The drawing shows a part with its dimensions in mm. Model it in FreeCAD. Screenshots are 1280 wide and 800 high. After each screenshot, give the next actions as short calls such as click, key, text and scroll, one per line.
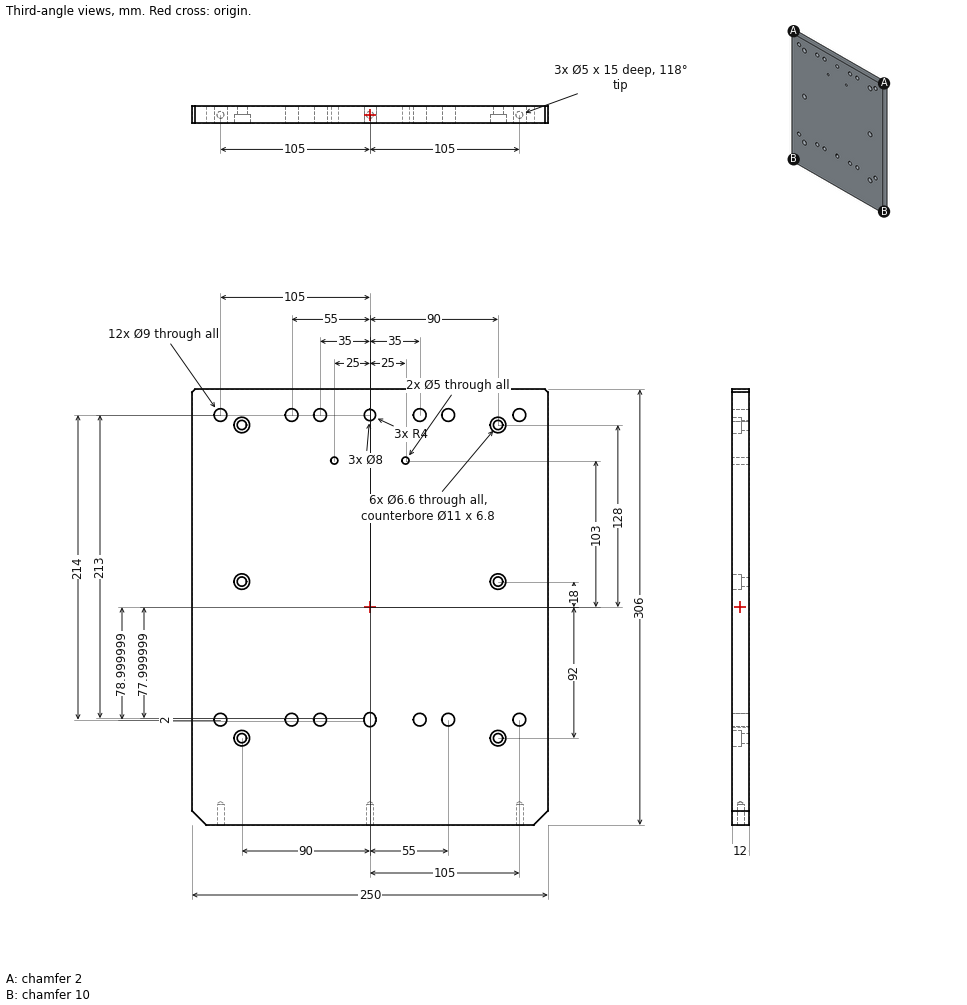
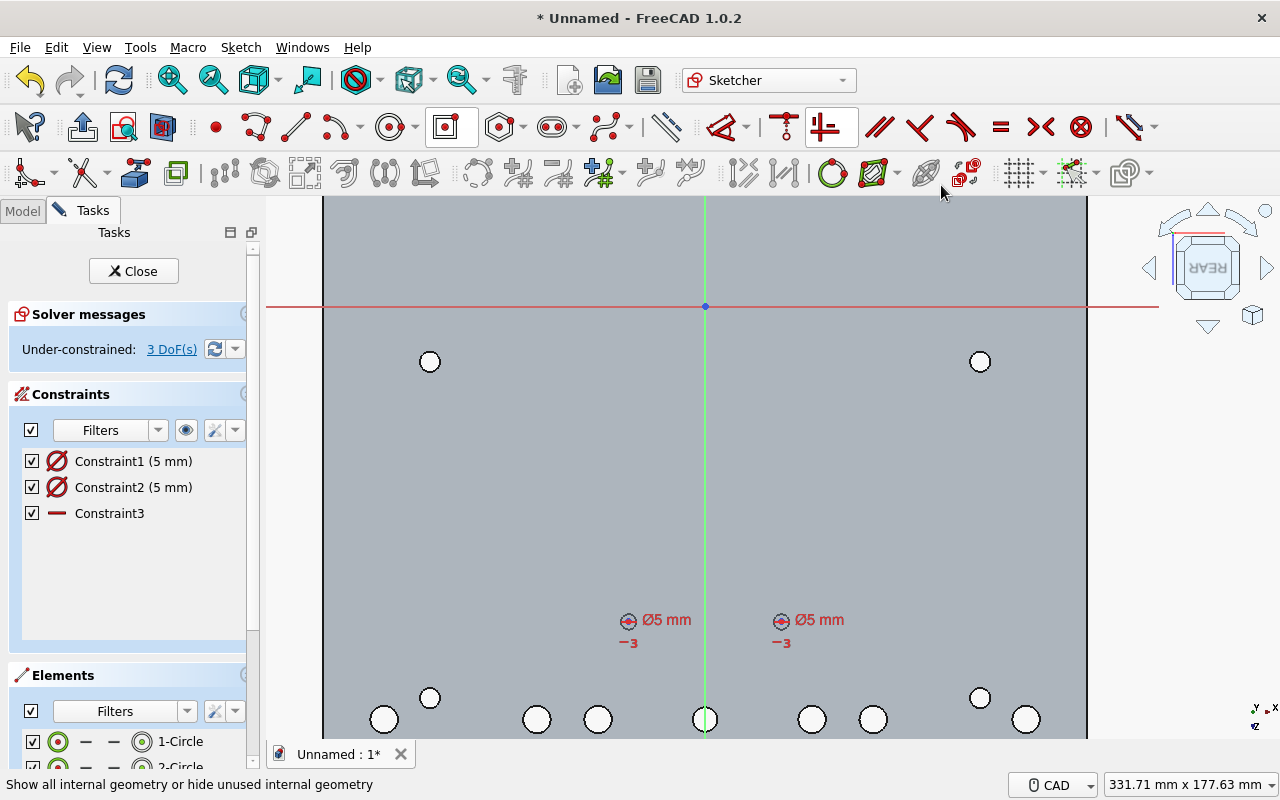
click(722, 128)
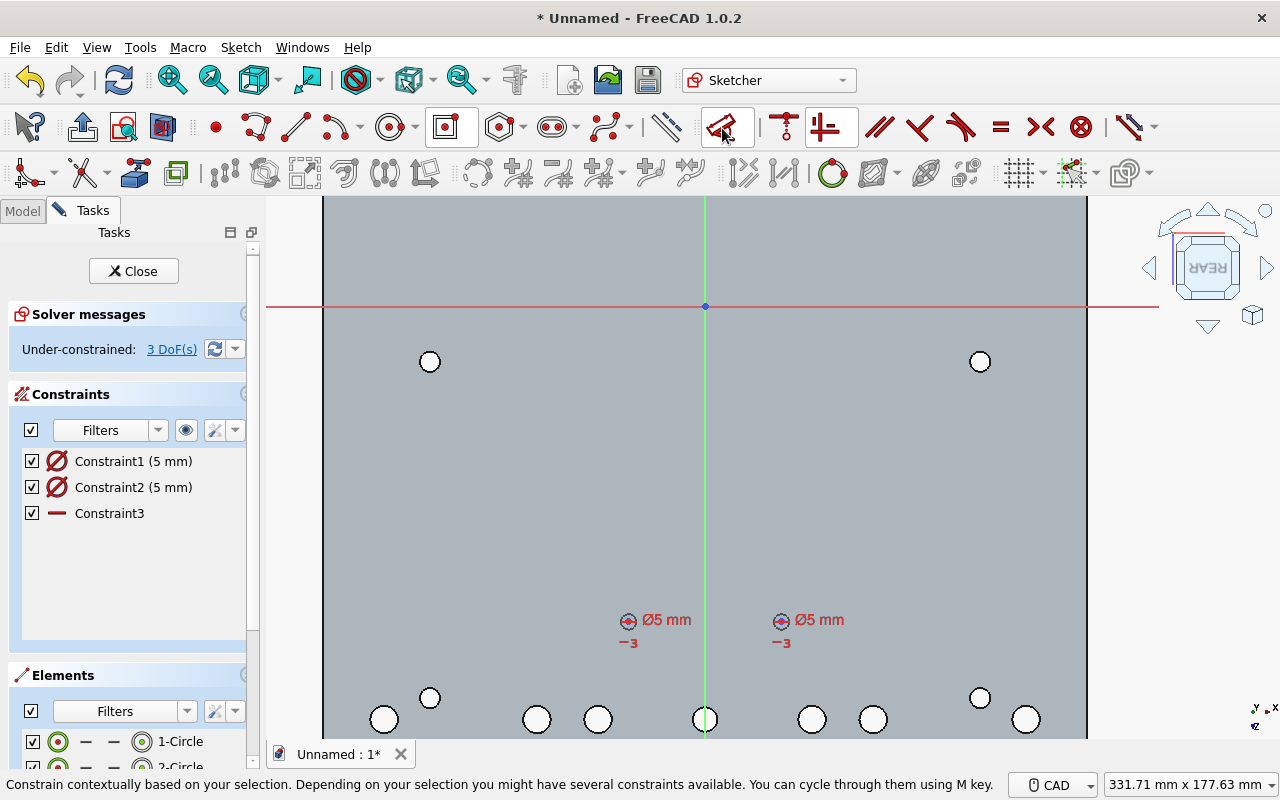
click(781, 622)
click(743, 273)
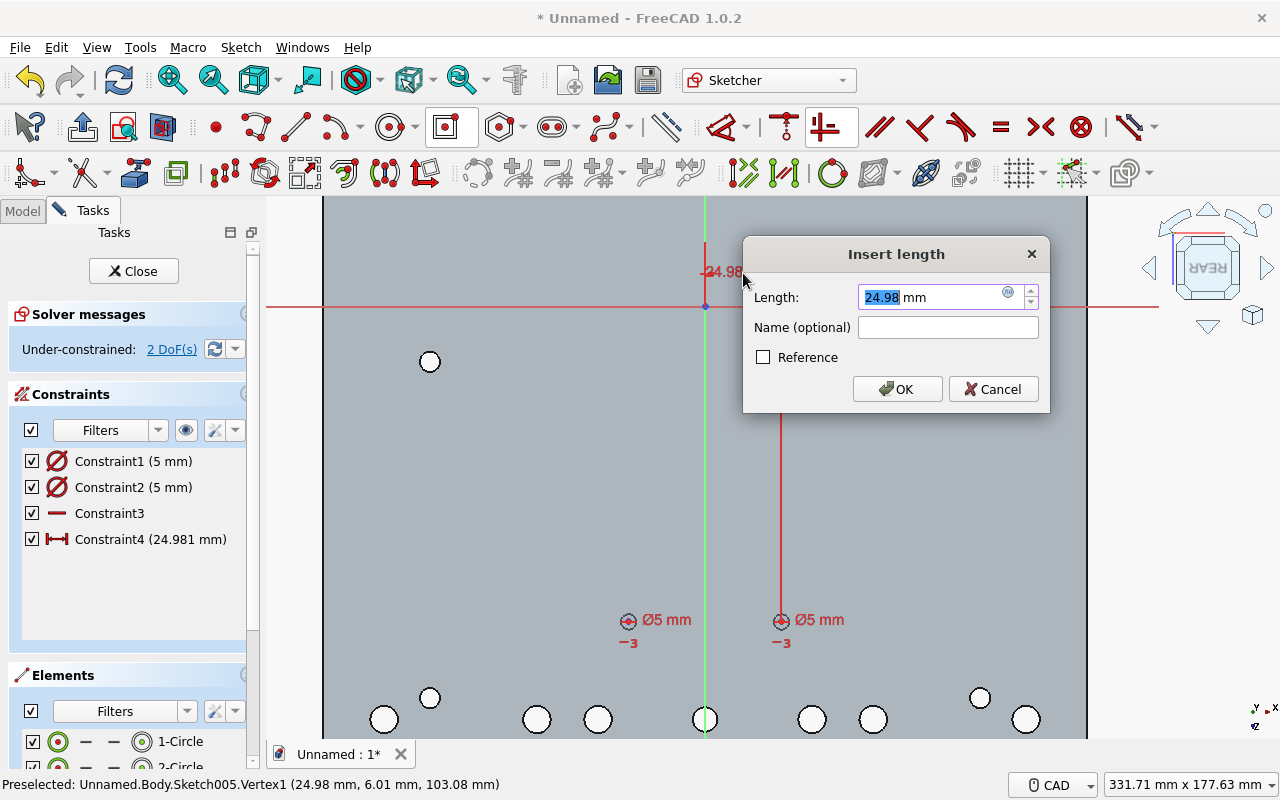
text(25)
key(Return)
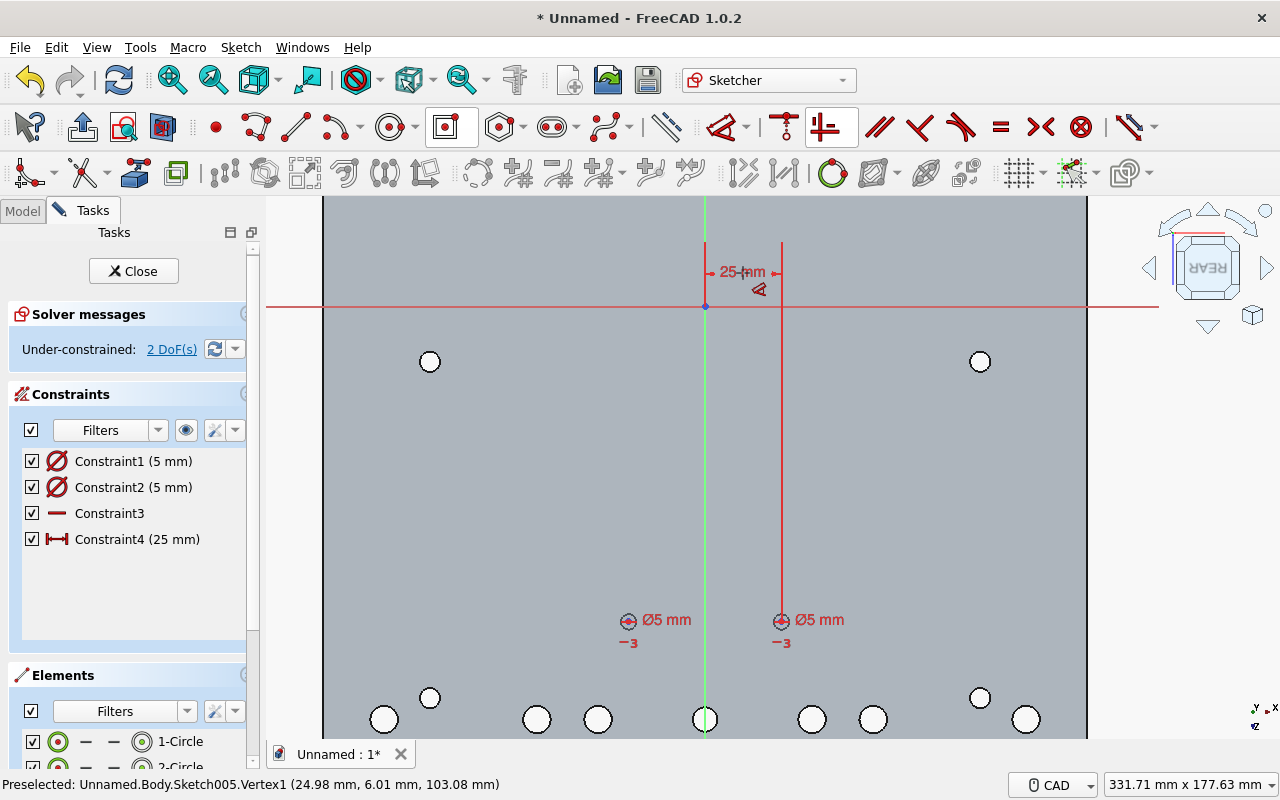
click(629, 622)
click(667, 273)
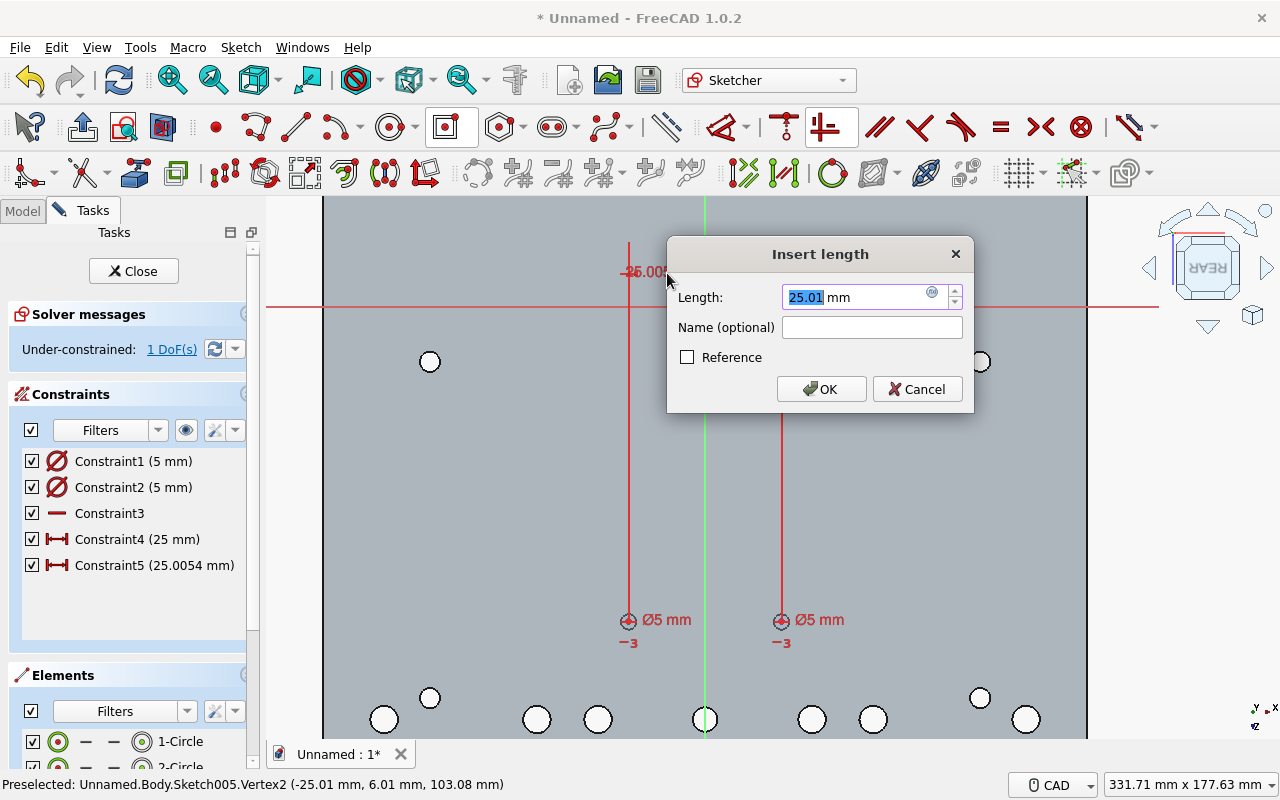
text(25)
key(Return)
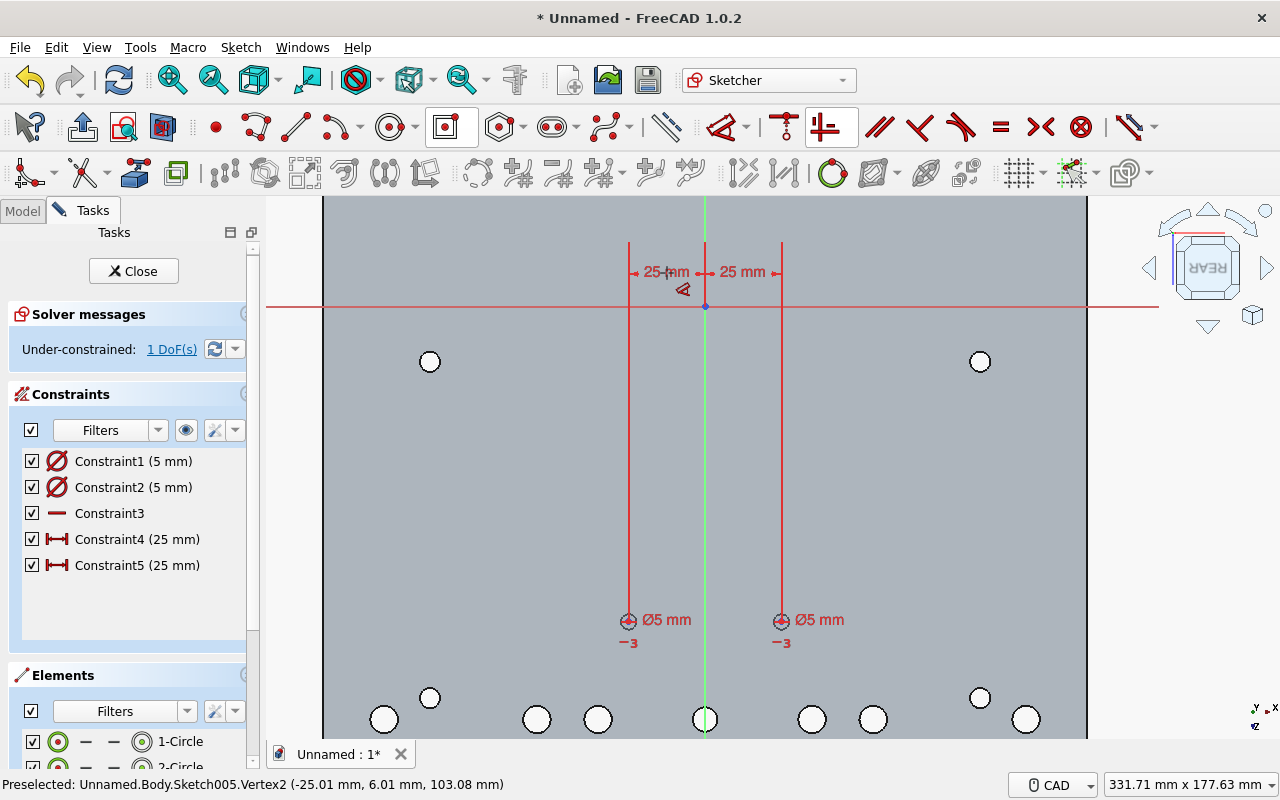
click(782, 622)
click(816, 464)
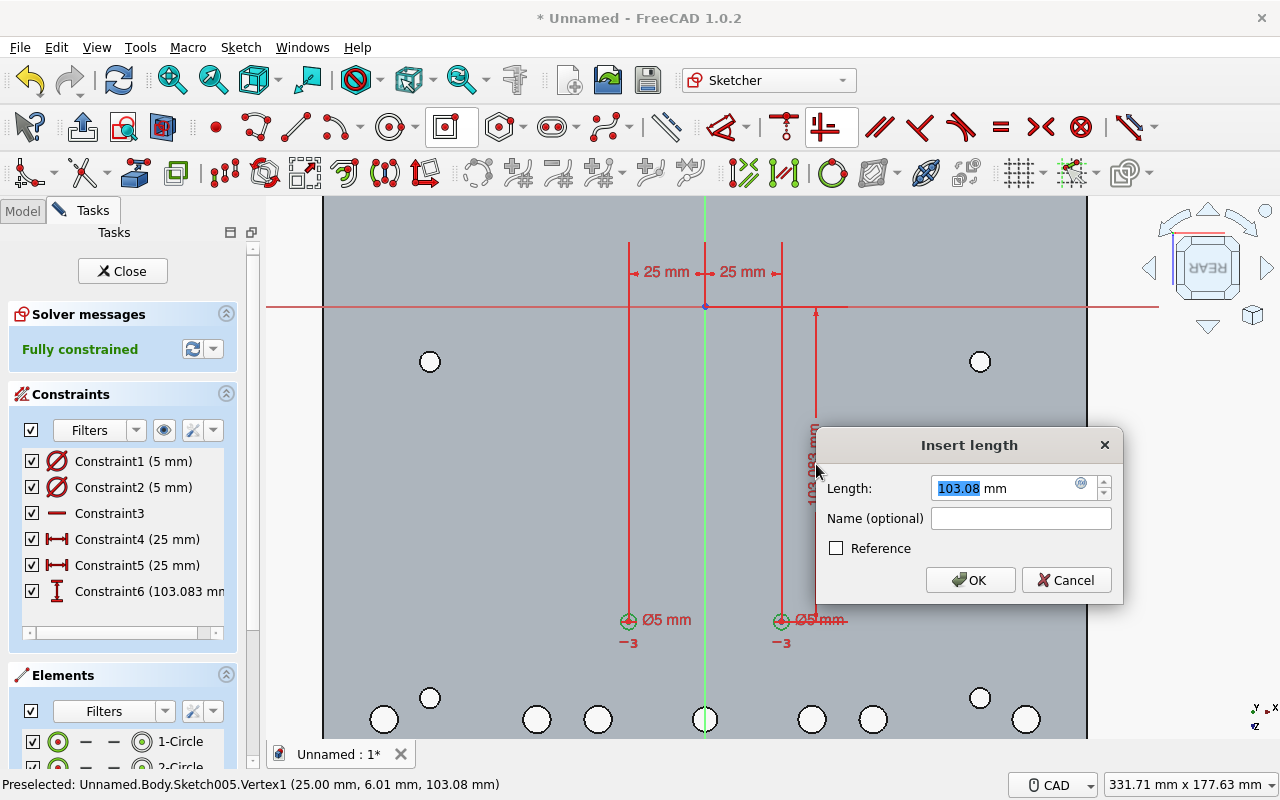
text(103)
key(Return)
key(Escape)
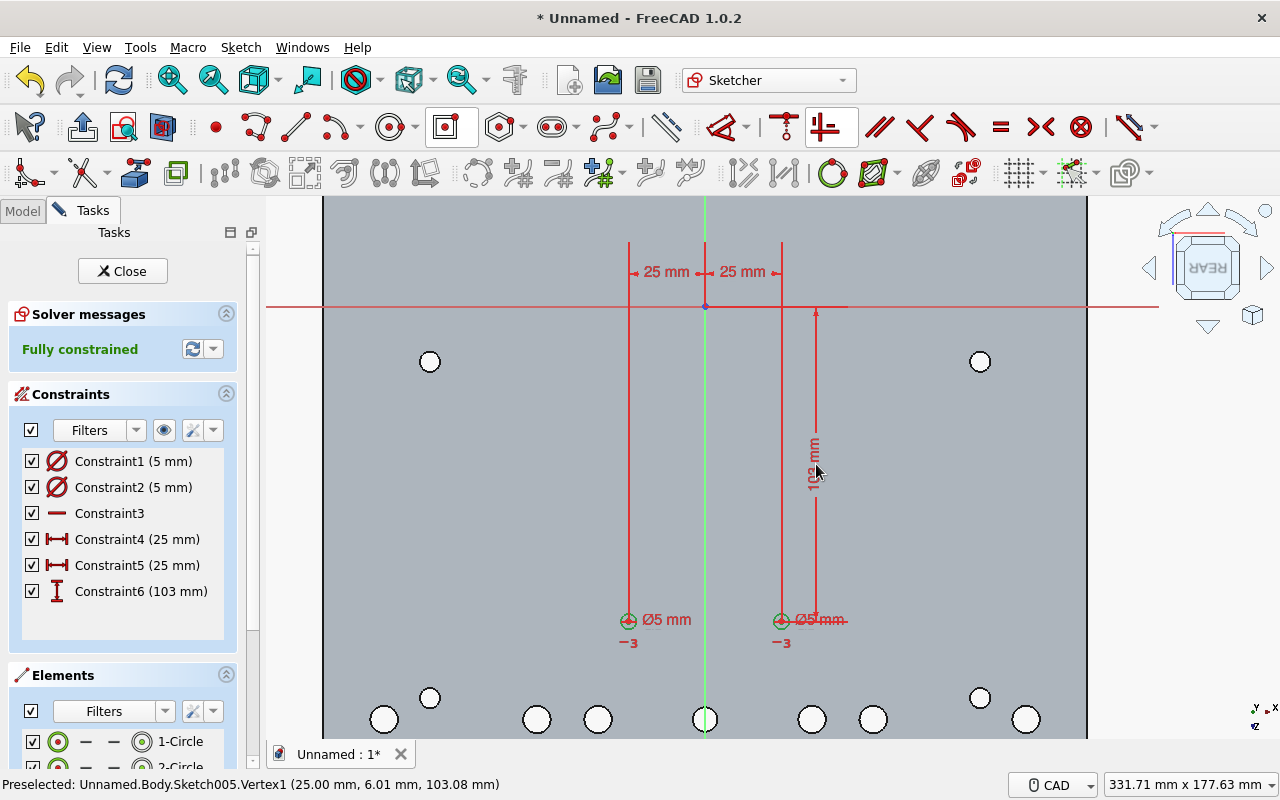
click(123, 271)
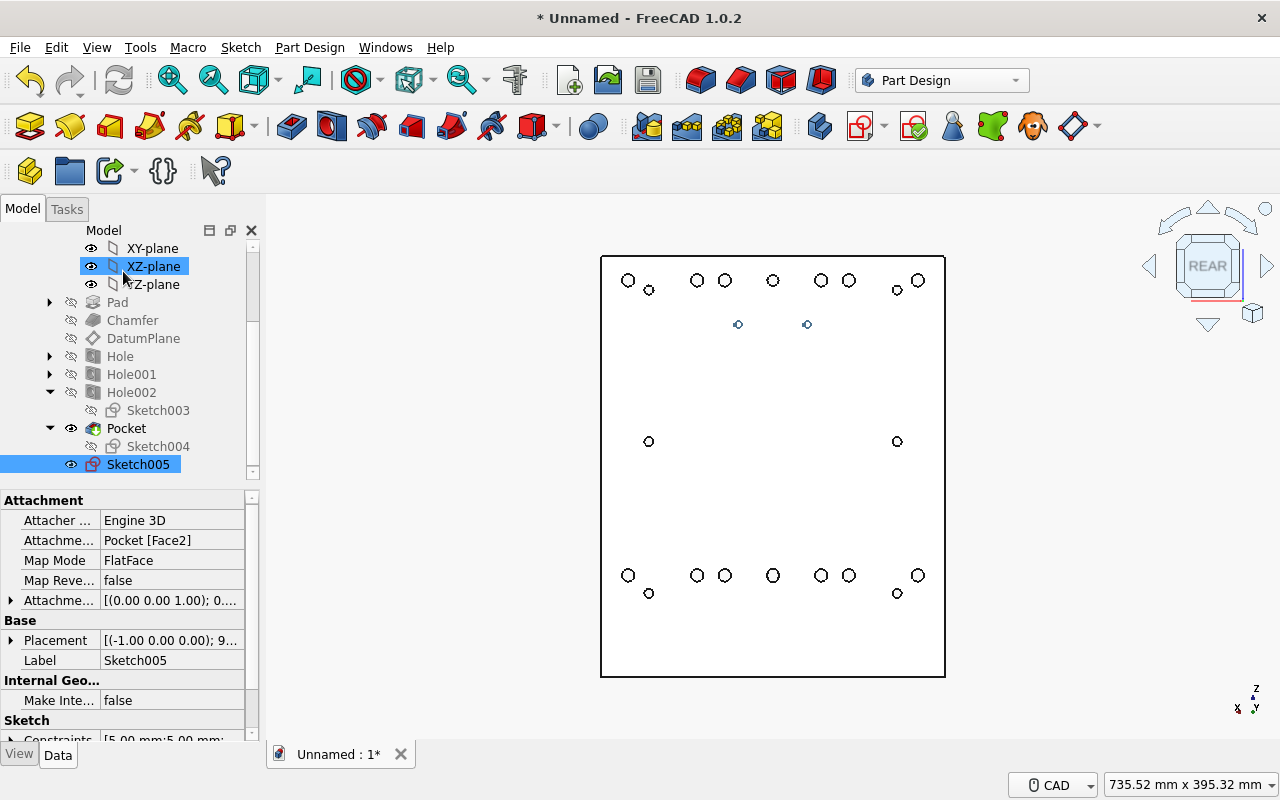
click(332, 126)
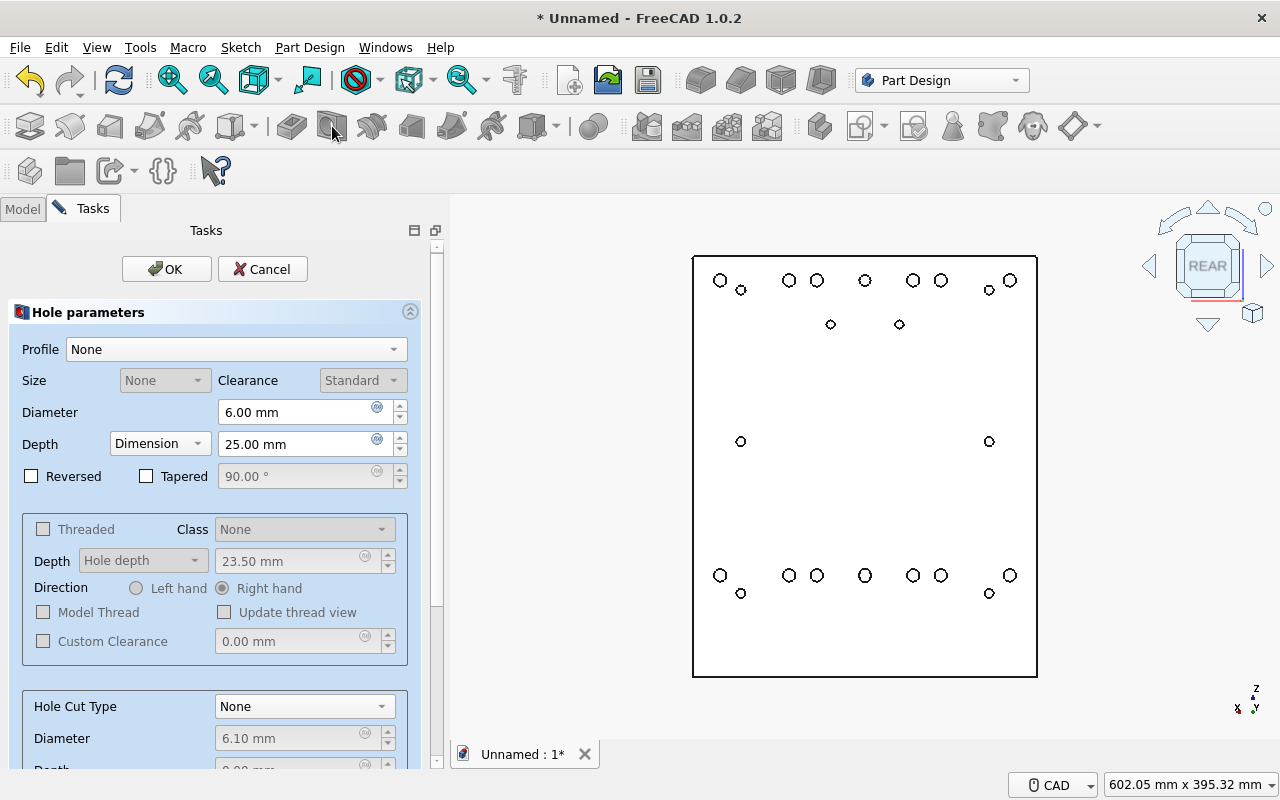
triple_click(305, 412)